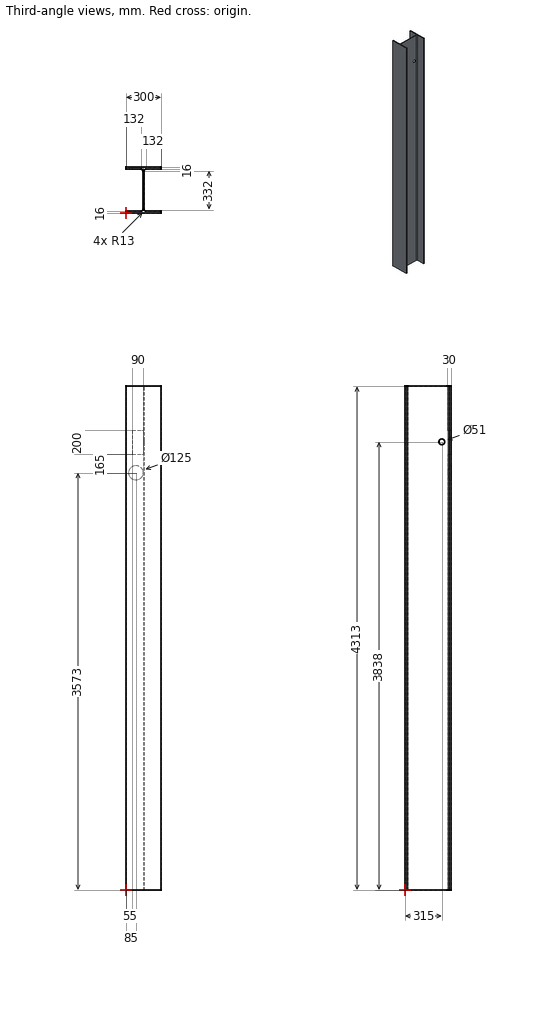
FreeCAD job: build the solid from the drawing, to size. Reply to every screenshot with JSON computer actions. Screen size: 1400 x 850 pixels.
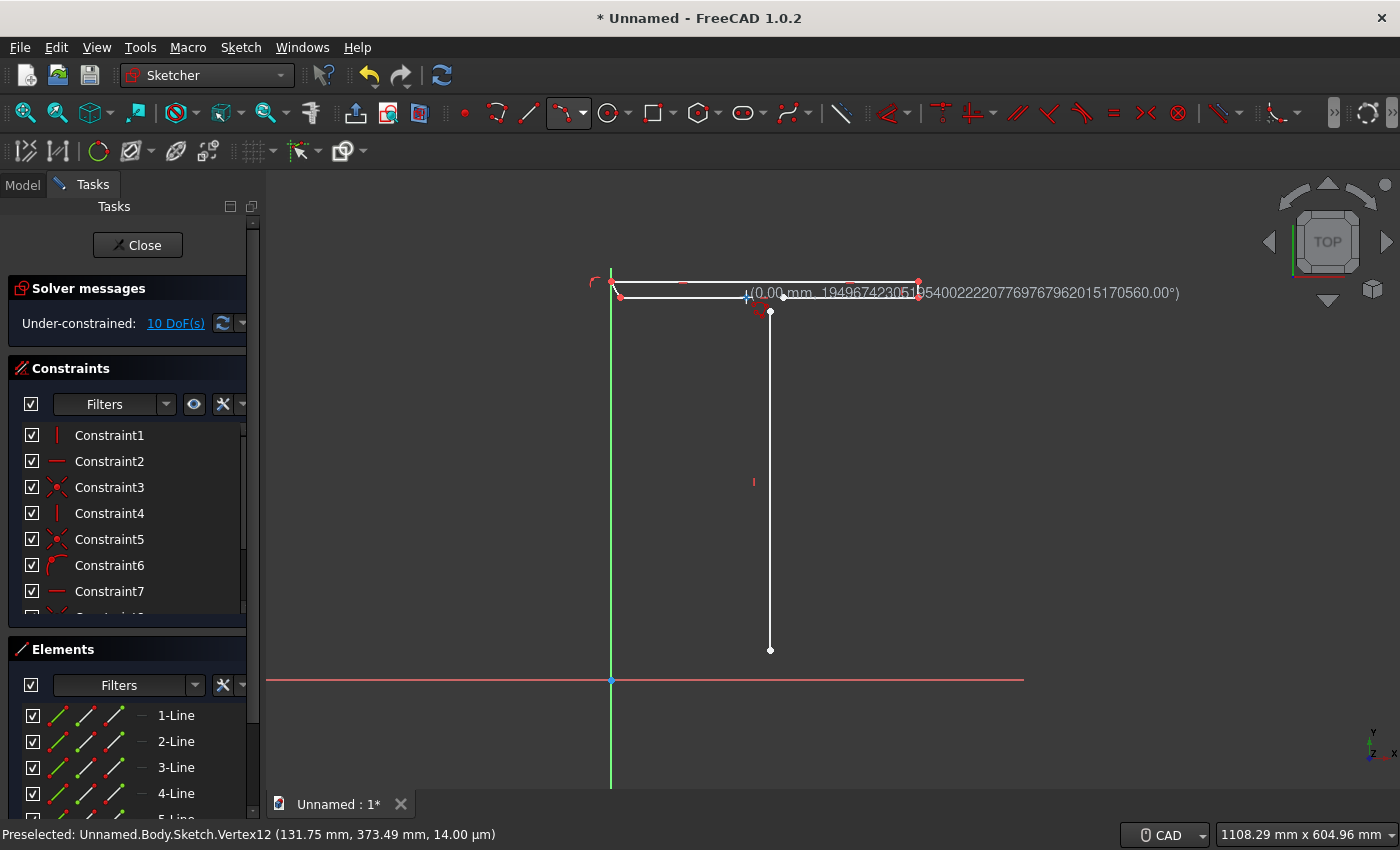
{"action": "key", "text": "g l"}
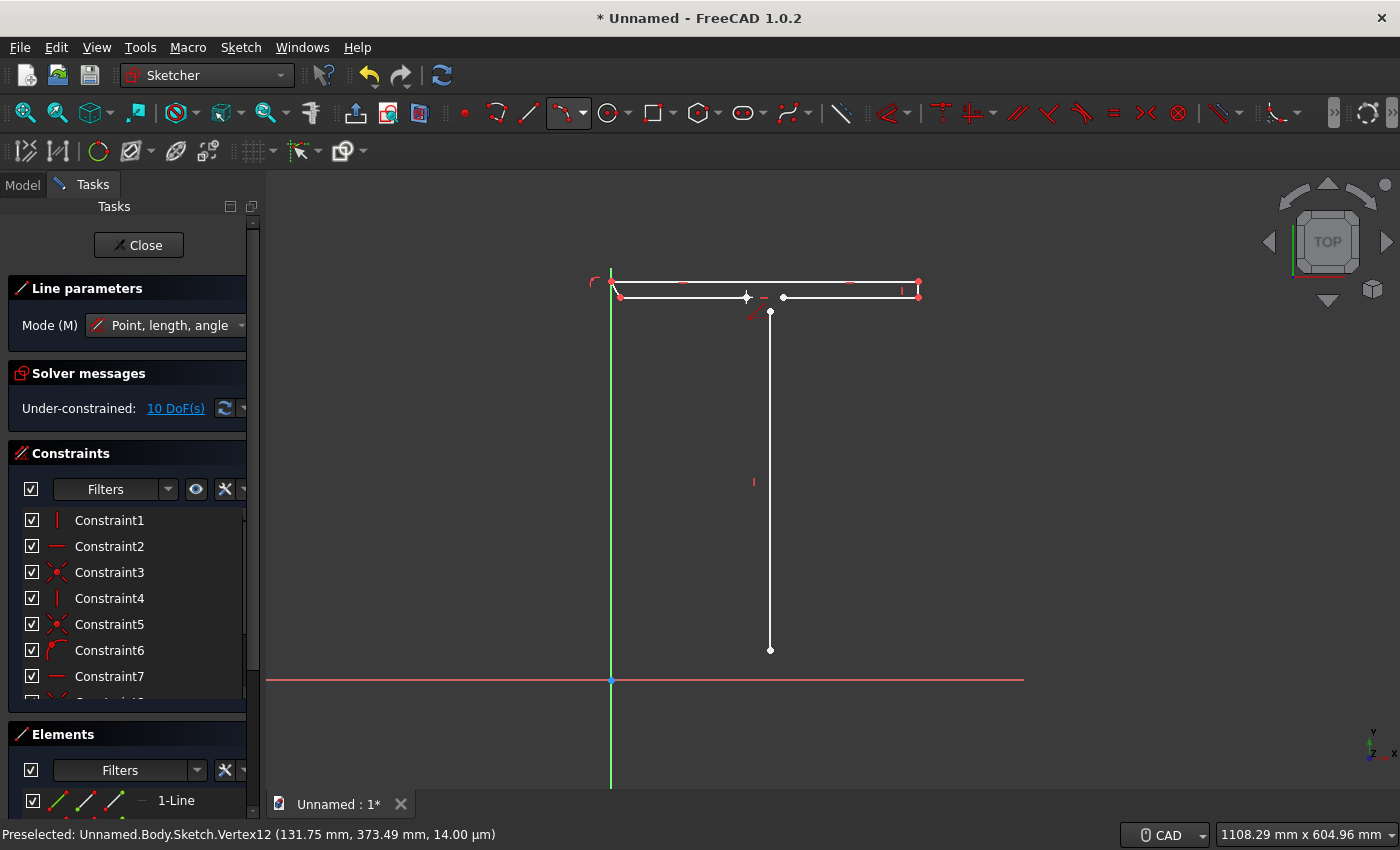
{"action": "scroll", "coordinate": [760, 311], "scroll_direction": "up", "scroll_amount": 3}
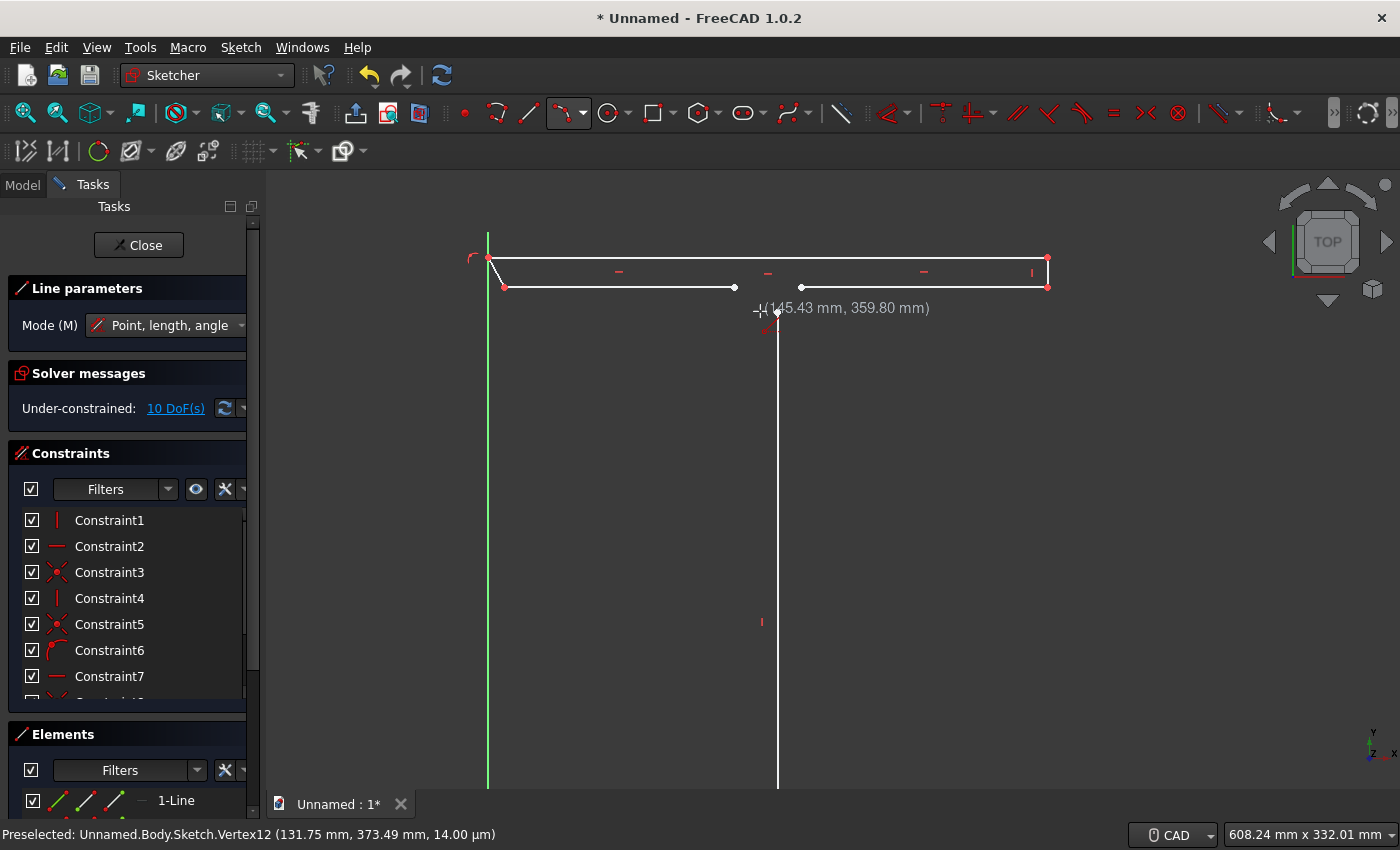
{"action": "left_click", "coordinate": [759, 310]}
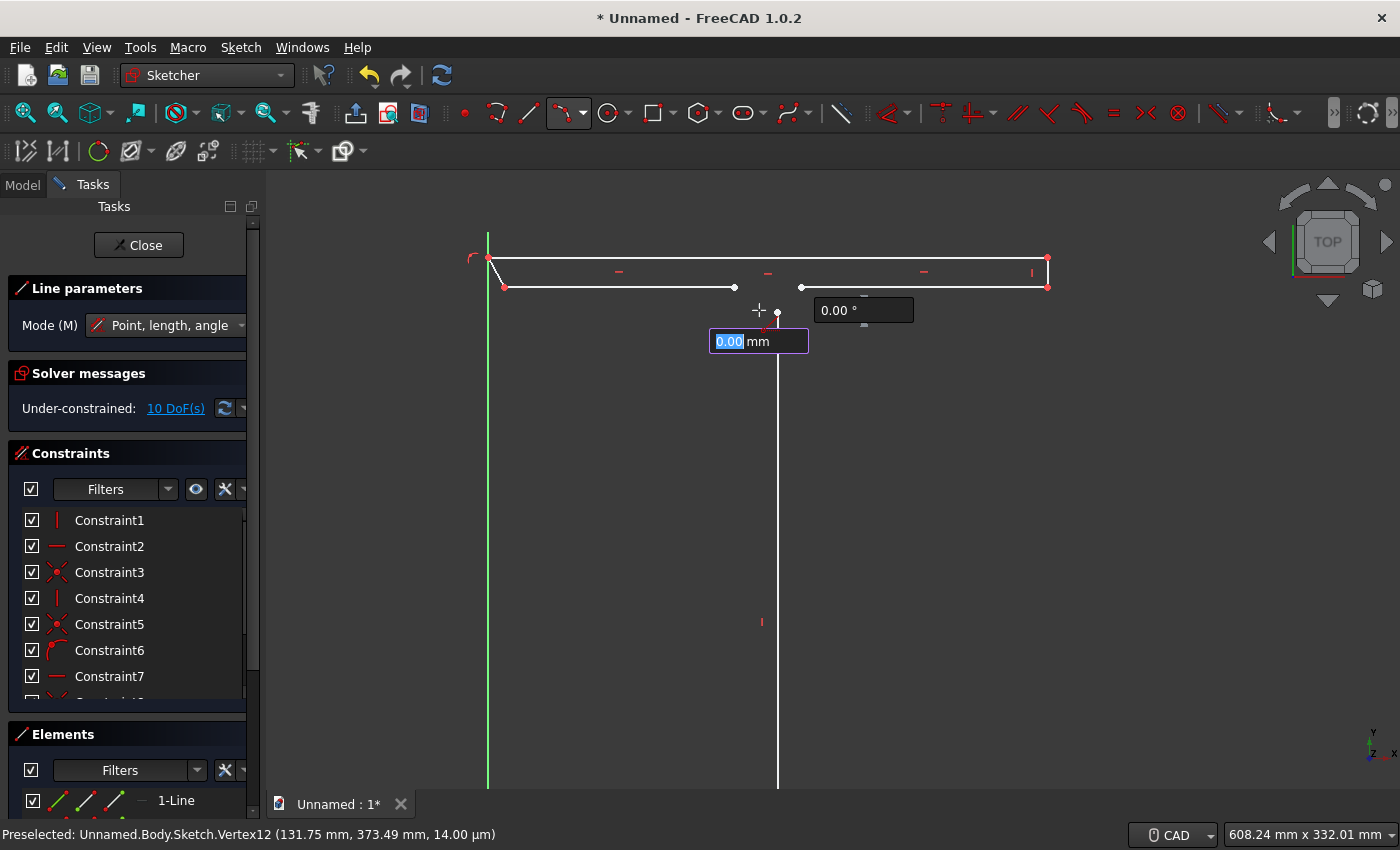
{"action": "scroll", "coordinate": [760, 309], "scroll_direction": "down", "scroll_amount": 3}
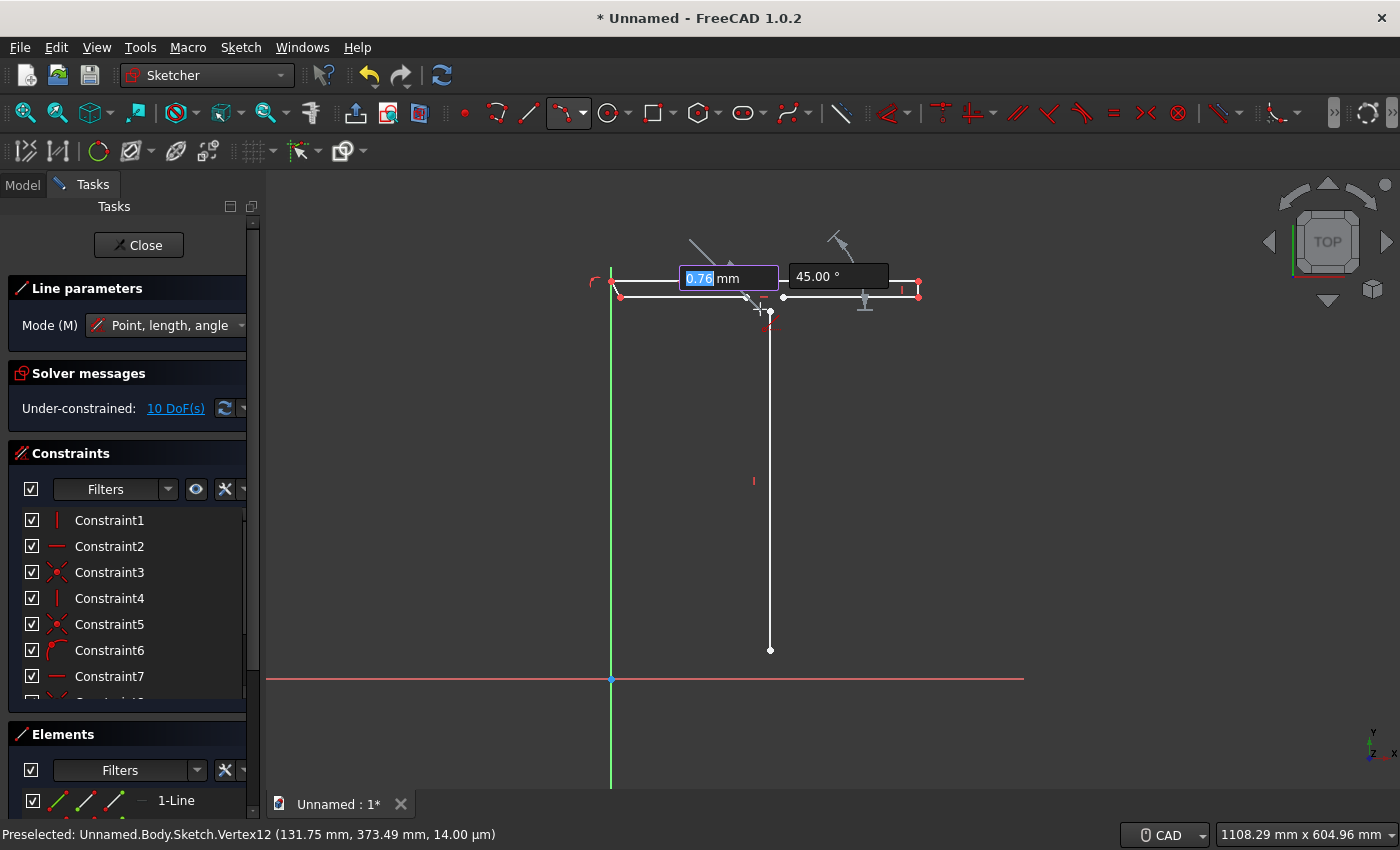
{"action": "scroll", "coordinate": [760, 650], "scroll_direction": "up", "scroll_amount": 3}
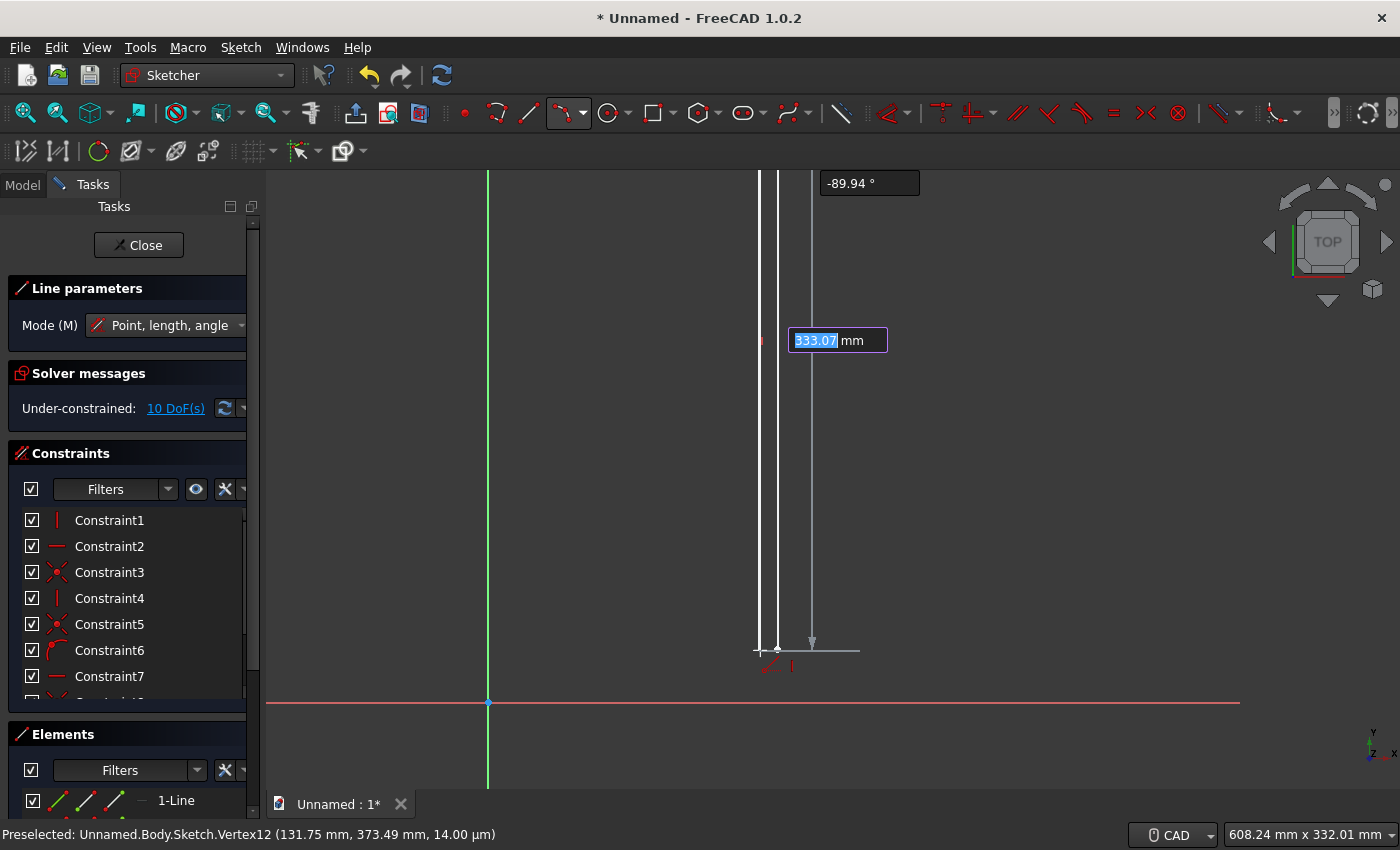
{"action": "left_click", "coordinate": [759, 649]}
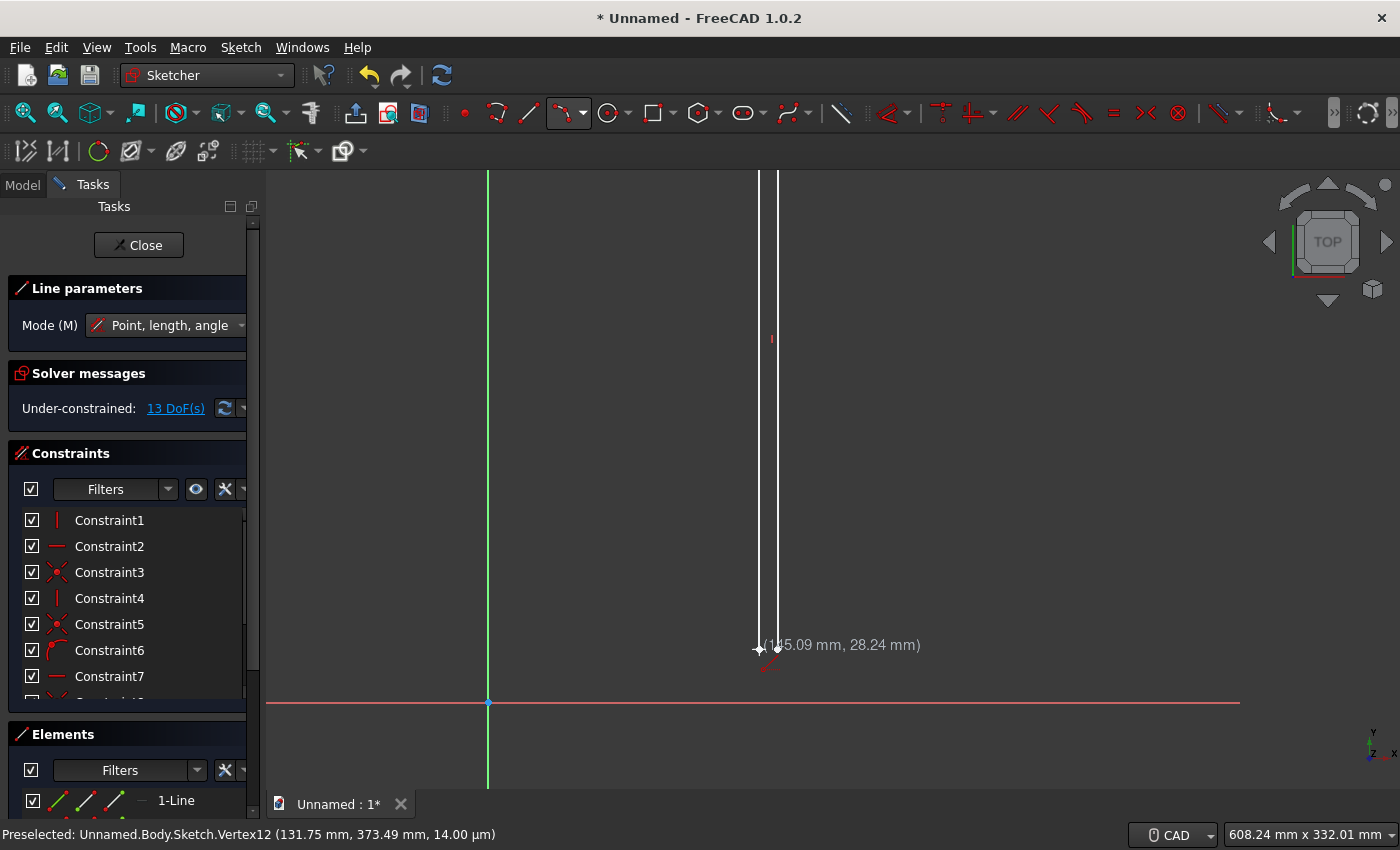
{"action": "left_click", "coordinate": [498, 114]}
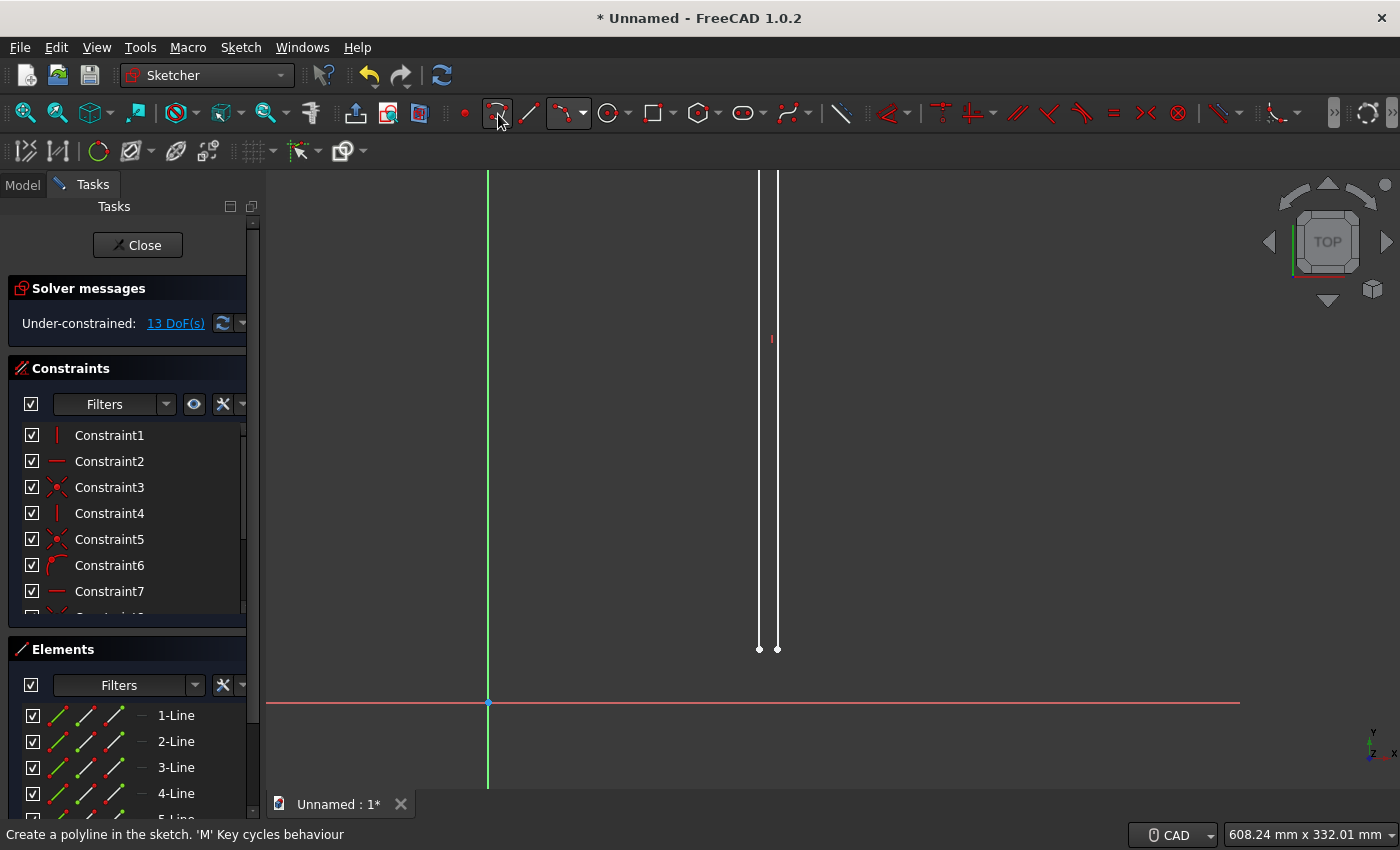
{"action": "left_click", "coordinate": [735, 673]}
{"action": "left_click", "coordinate": [488, 673]}
{"action": "left_click", "coordinate": [488, 703]}
{"action": "left_click", "coordinate": [1048, 694]}
{"action": "left_click", "coordinate": [1048, 673]}
{"action": "left_click", "coordinate": [802, 673]}
{"action": "right_click", "coordinate": [802, 673]}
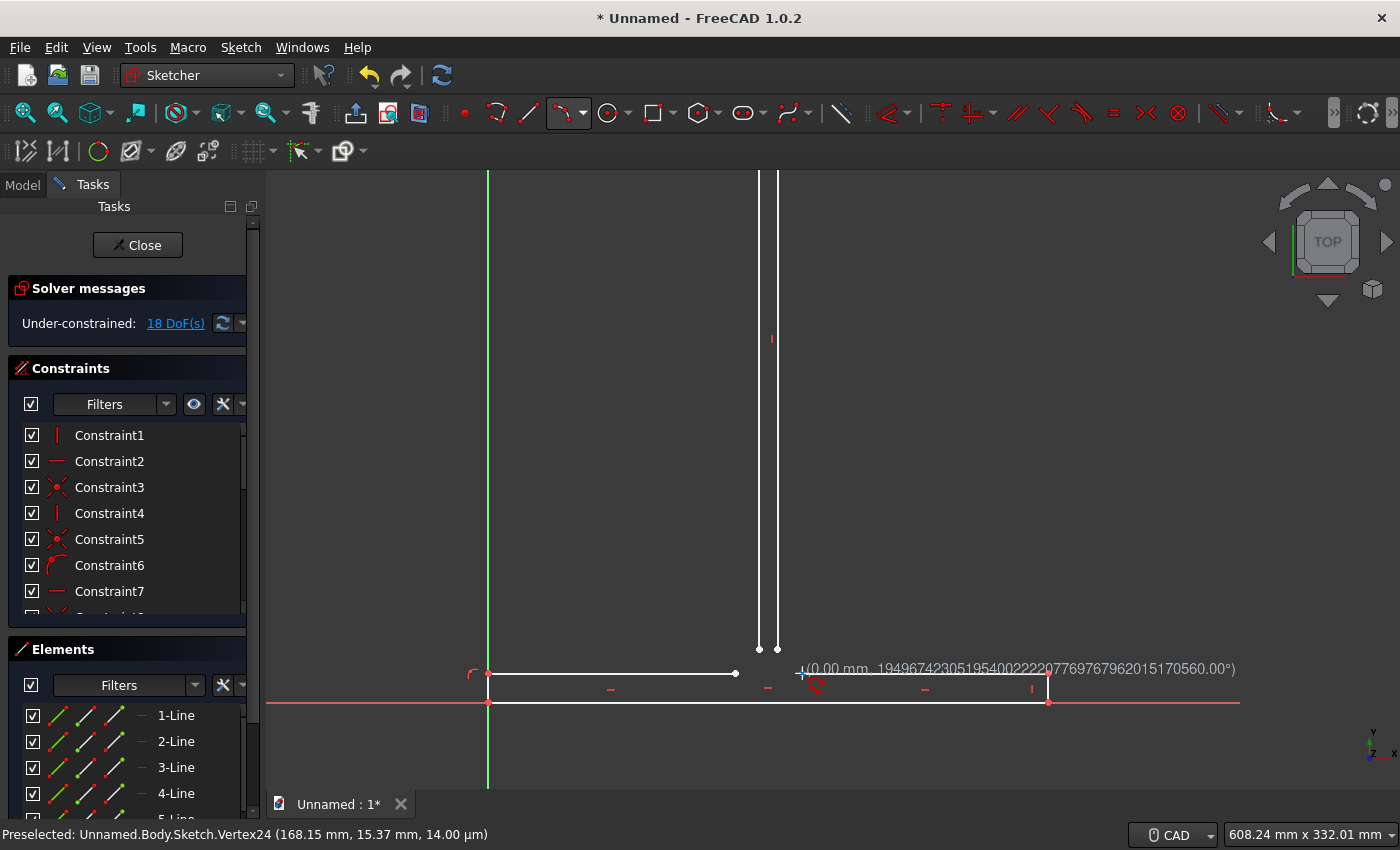
{"action": "left_click", "coordinate": [562, 114]}